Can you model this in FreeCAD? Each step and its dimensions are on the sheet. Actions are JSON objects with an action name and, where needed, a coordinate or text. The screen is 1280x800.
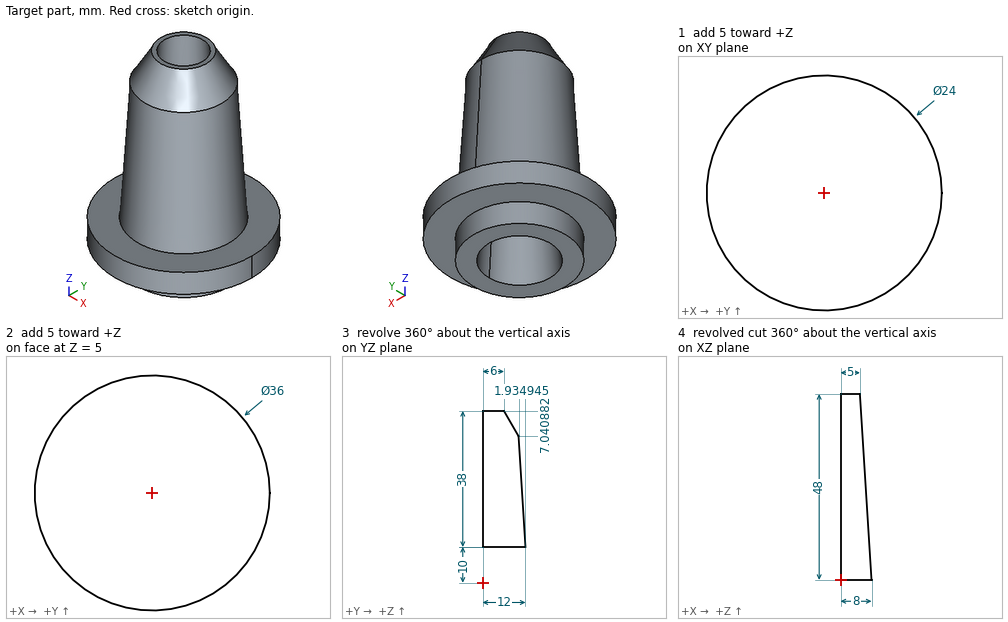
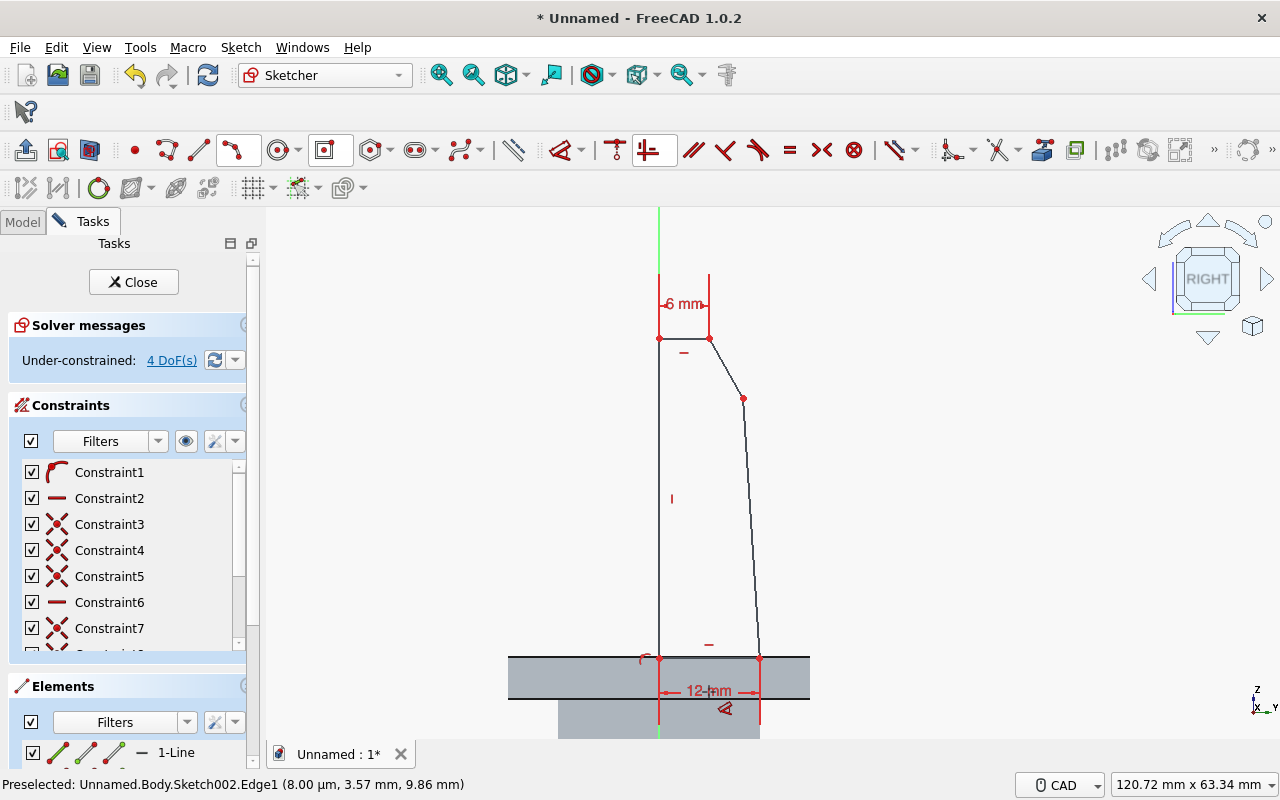
{"action": "left_click", "coordinate": [659, 435]}
{"action": "left_click", "coordinate": [625, 499]}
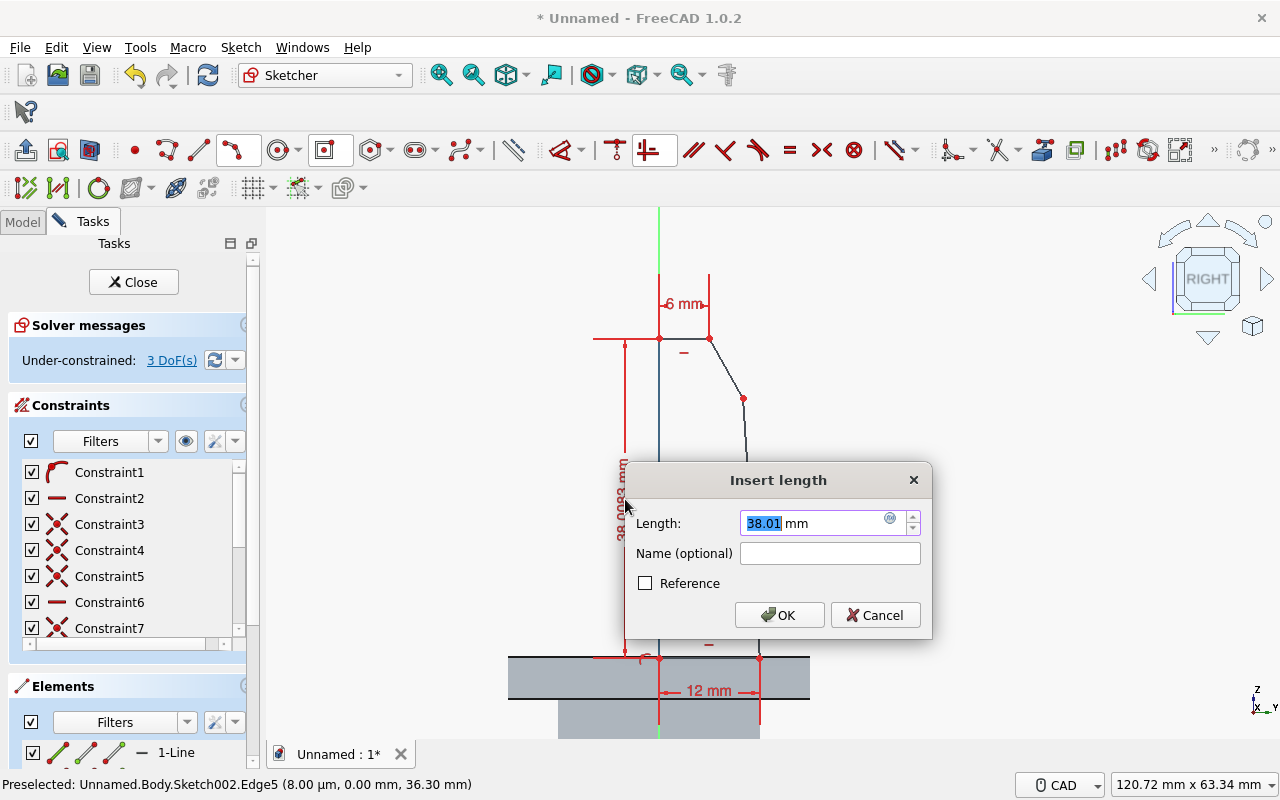
{"action": "type", "text": "38"}
{"action": "key", "text": "Return"}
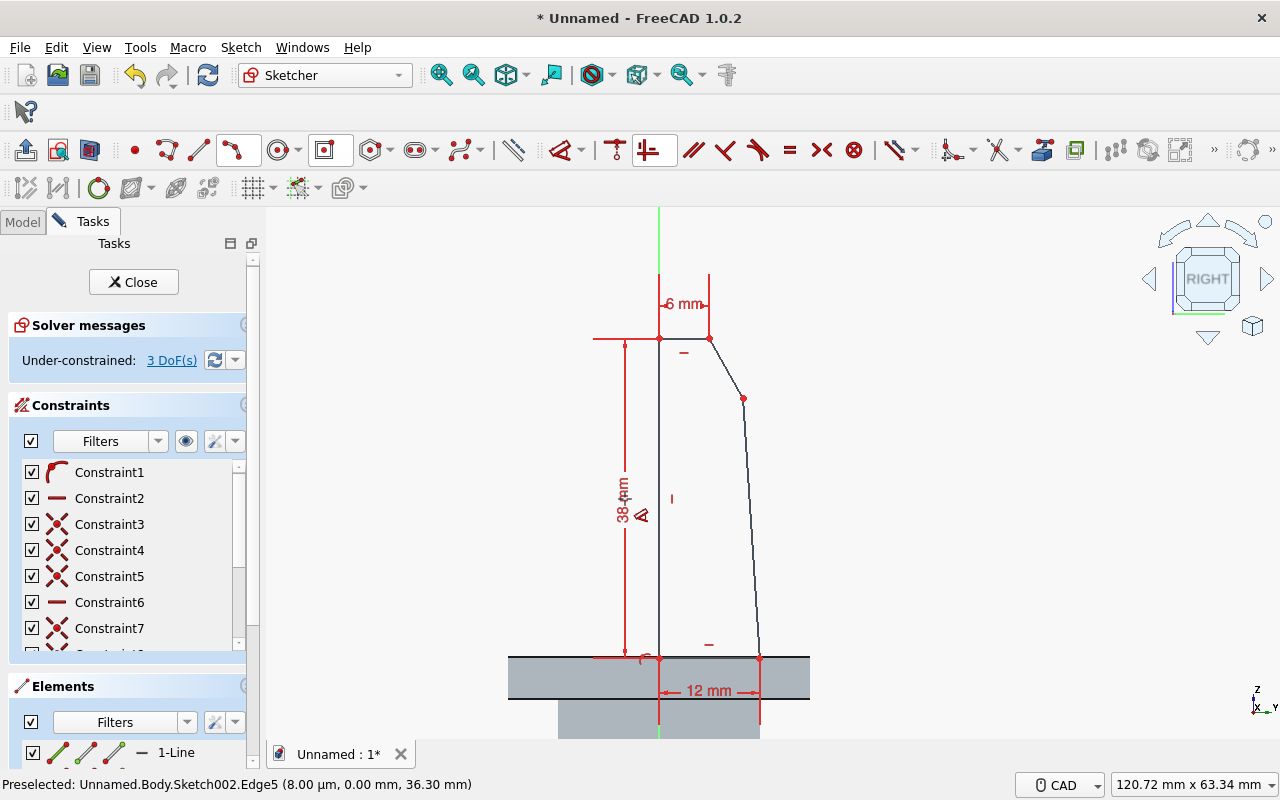
{"action": "left_click", "coordinate": [659, 658]}
{"action": "left_click", "coordinate": [625, 685]}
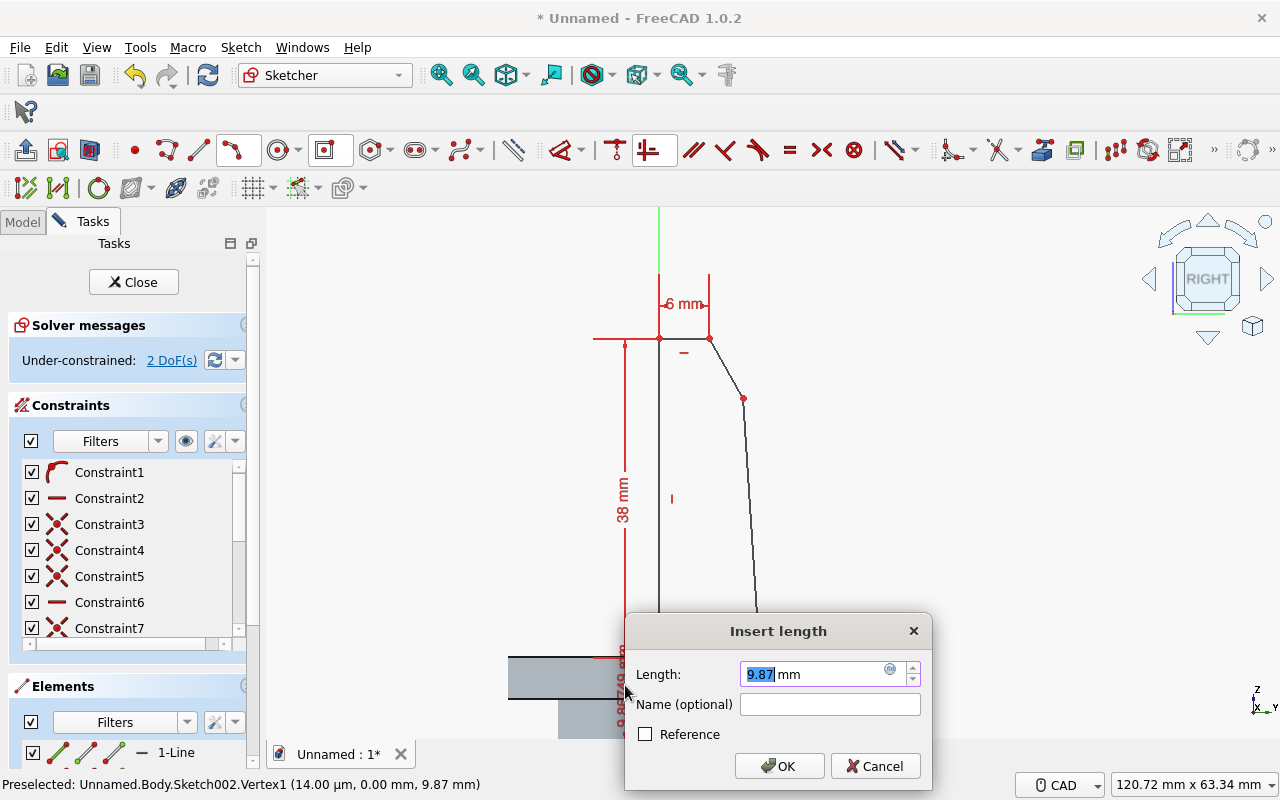
{"action": "type", "text": "10"}
{"action": "key", "text": "Return"}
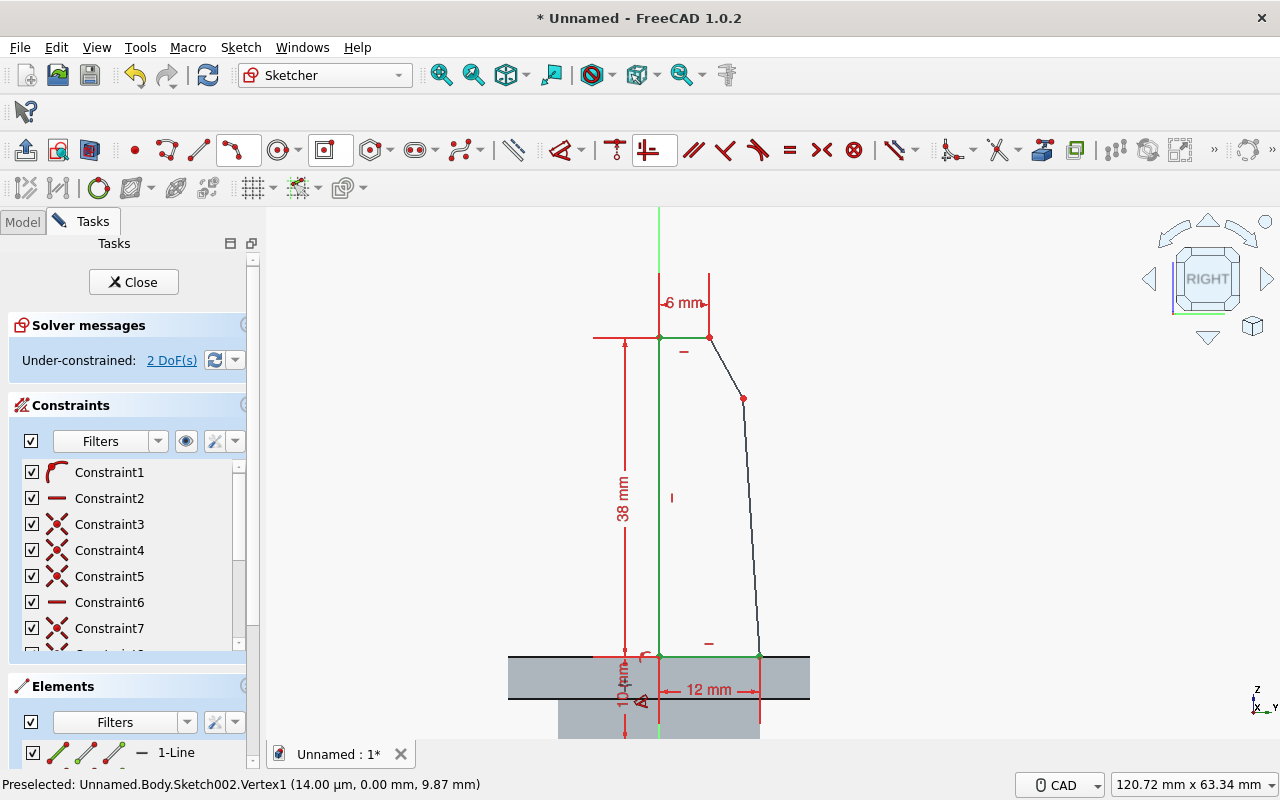
{"action": "scroll", "coordinate": [755, 579], "scroll_direction": "up", "scroll_amount": 5}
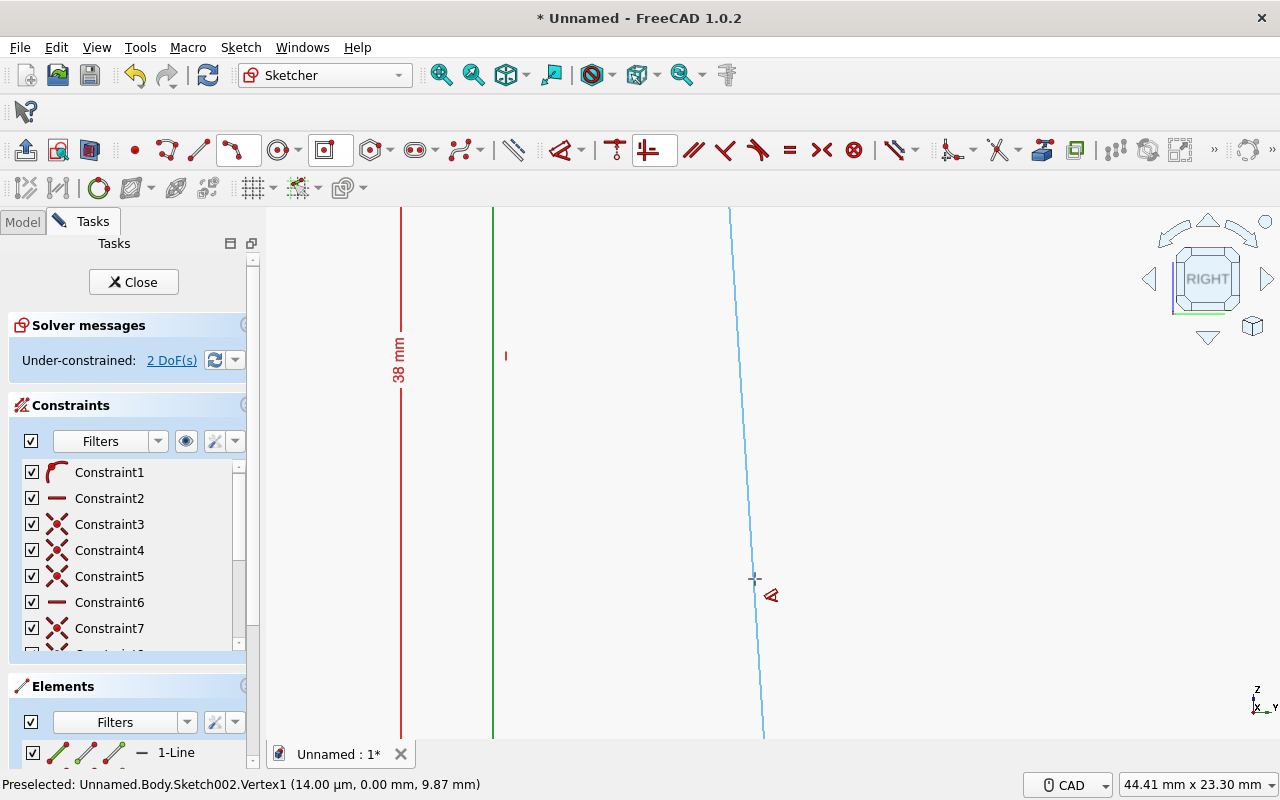
{"action": "left_click", "coordinate": [754, 579]}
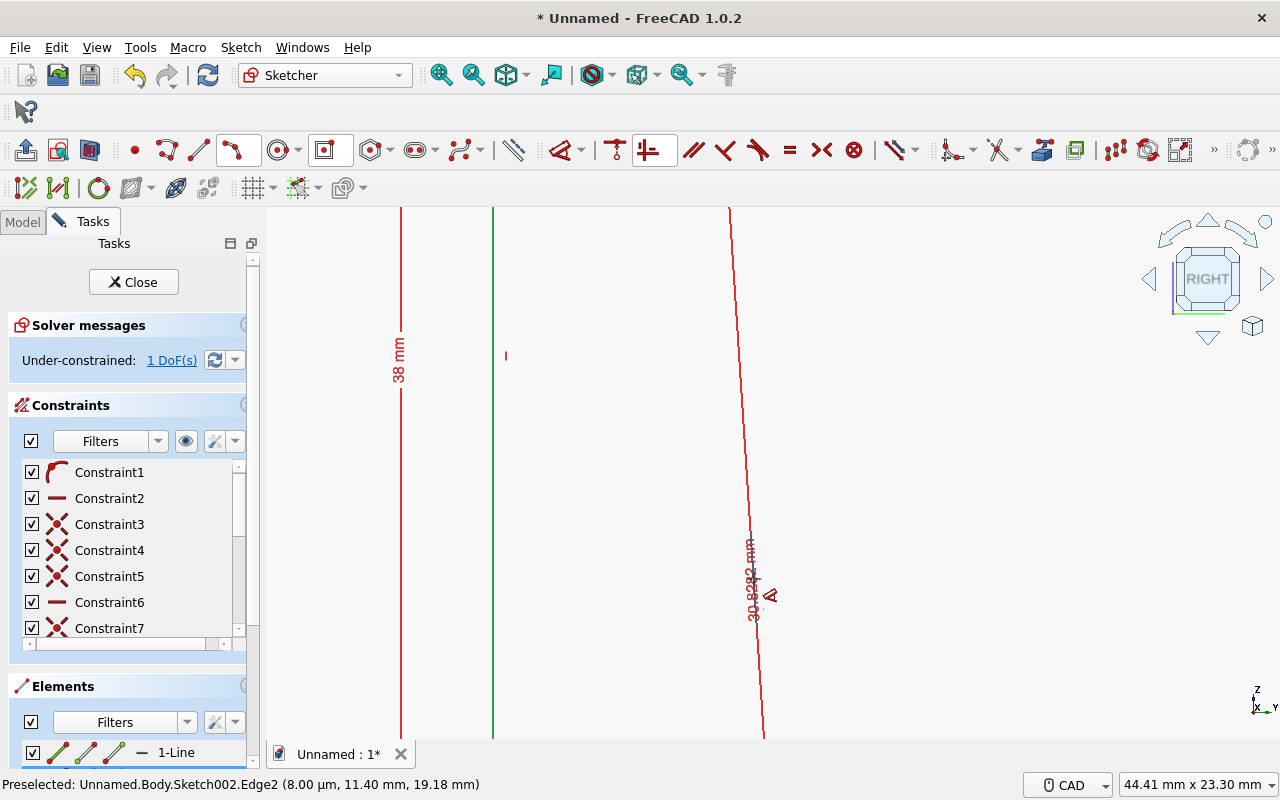
{"action": "key", "text": "Escape"}
{"action": "key", "text": "Escape"}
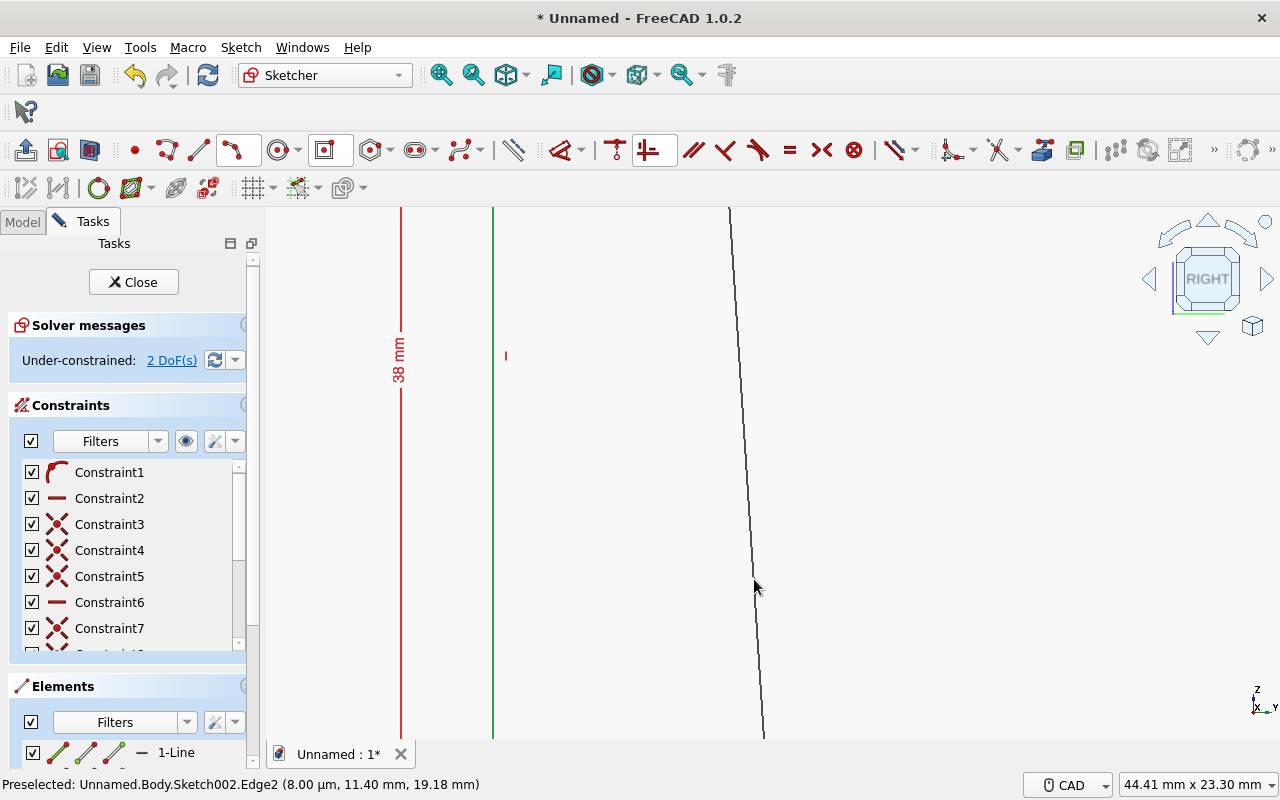
{"action": "left_click", "coordinate": [754, 579]}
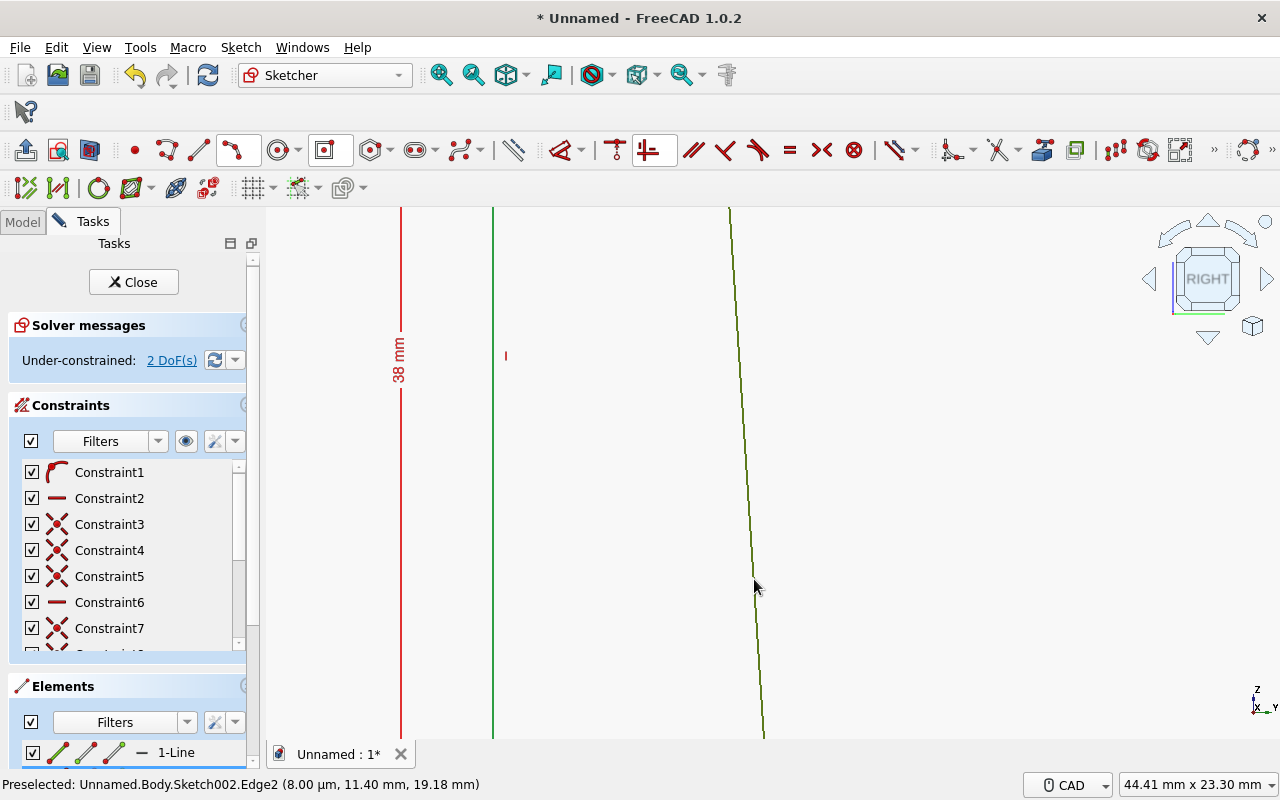
{"action": "left_click", "coordinate": [584, 150]}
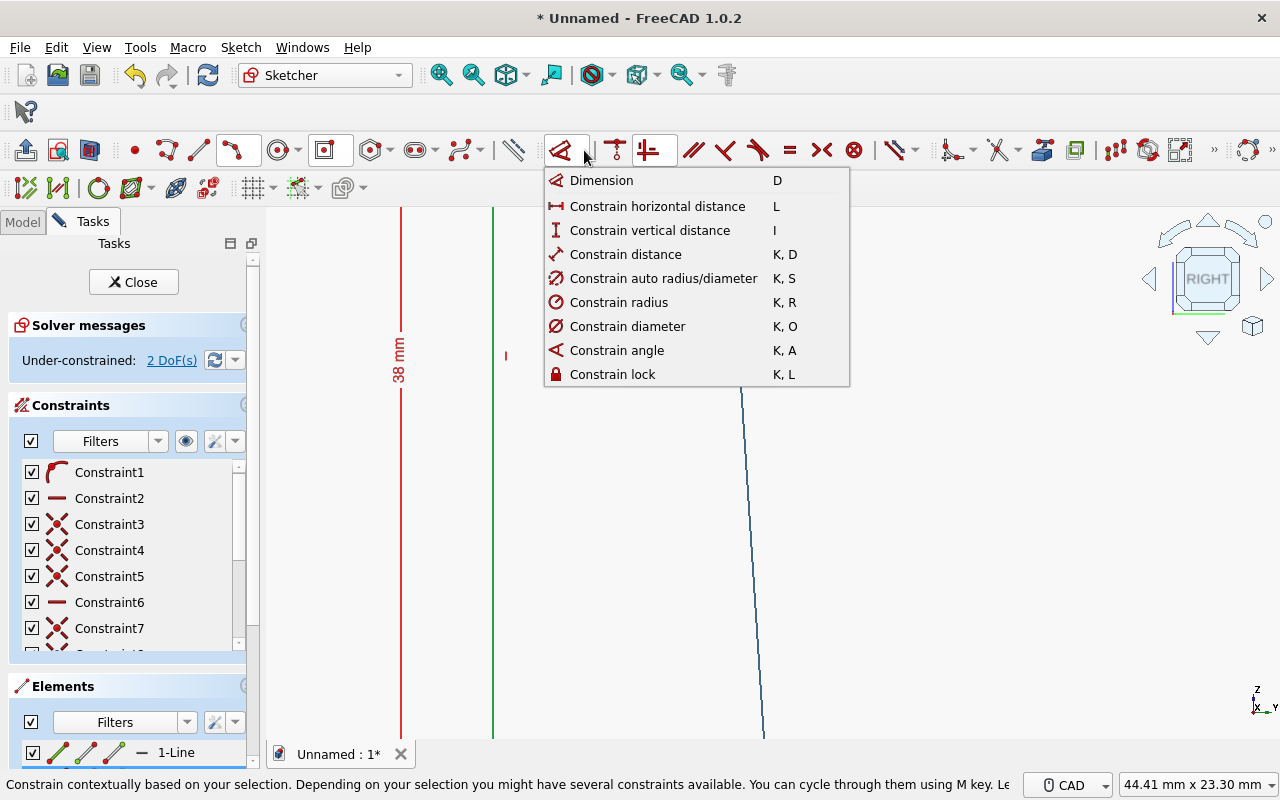
{"action": "left_click", "coordinate": [697, 206]}